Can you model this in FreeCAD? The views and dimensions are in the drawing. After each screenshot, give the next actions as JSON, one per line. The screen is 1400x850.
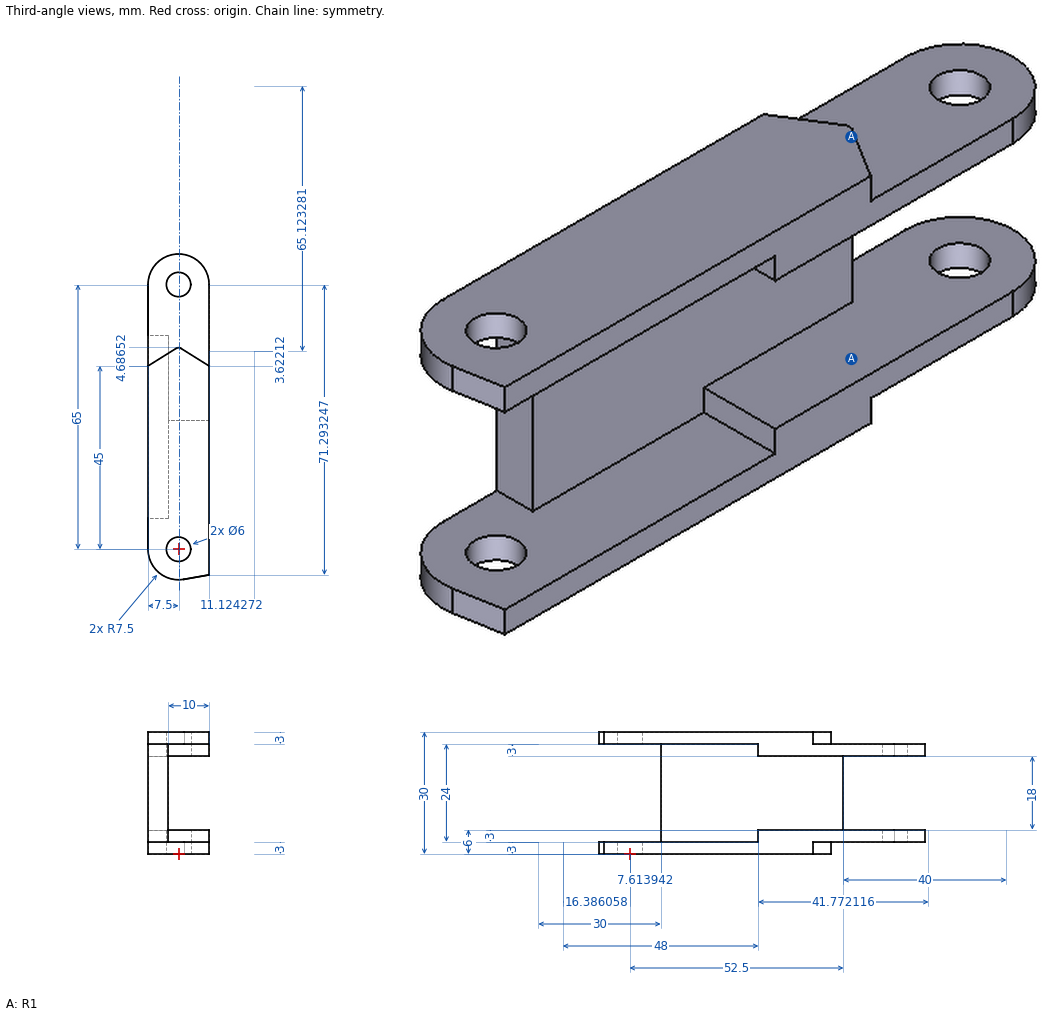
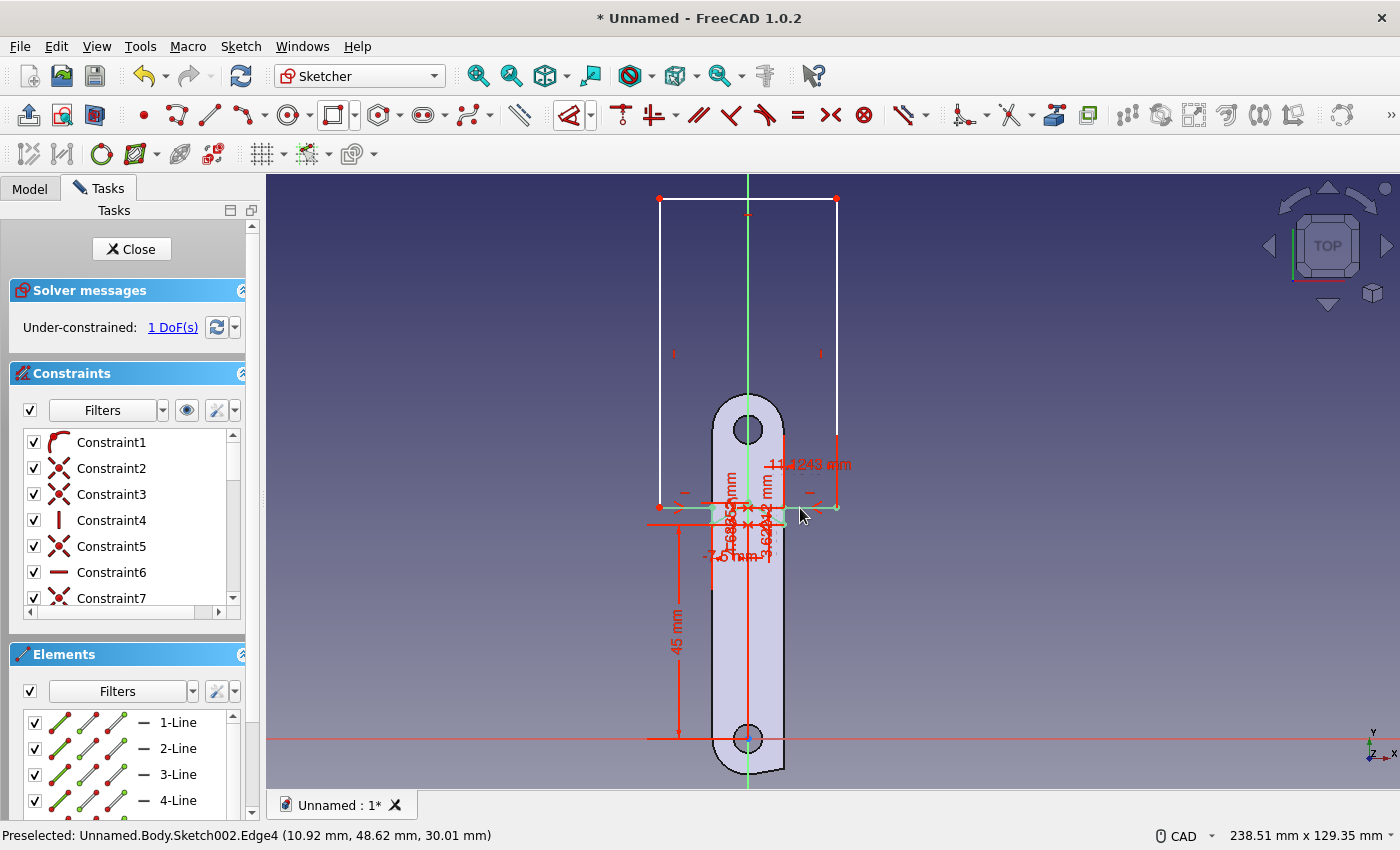
{"action": "left_click", "coordinate": [837, 415]}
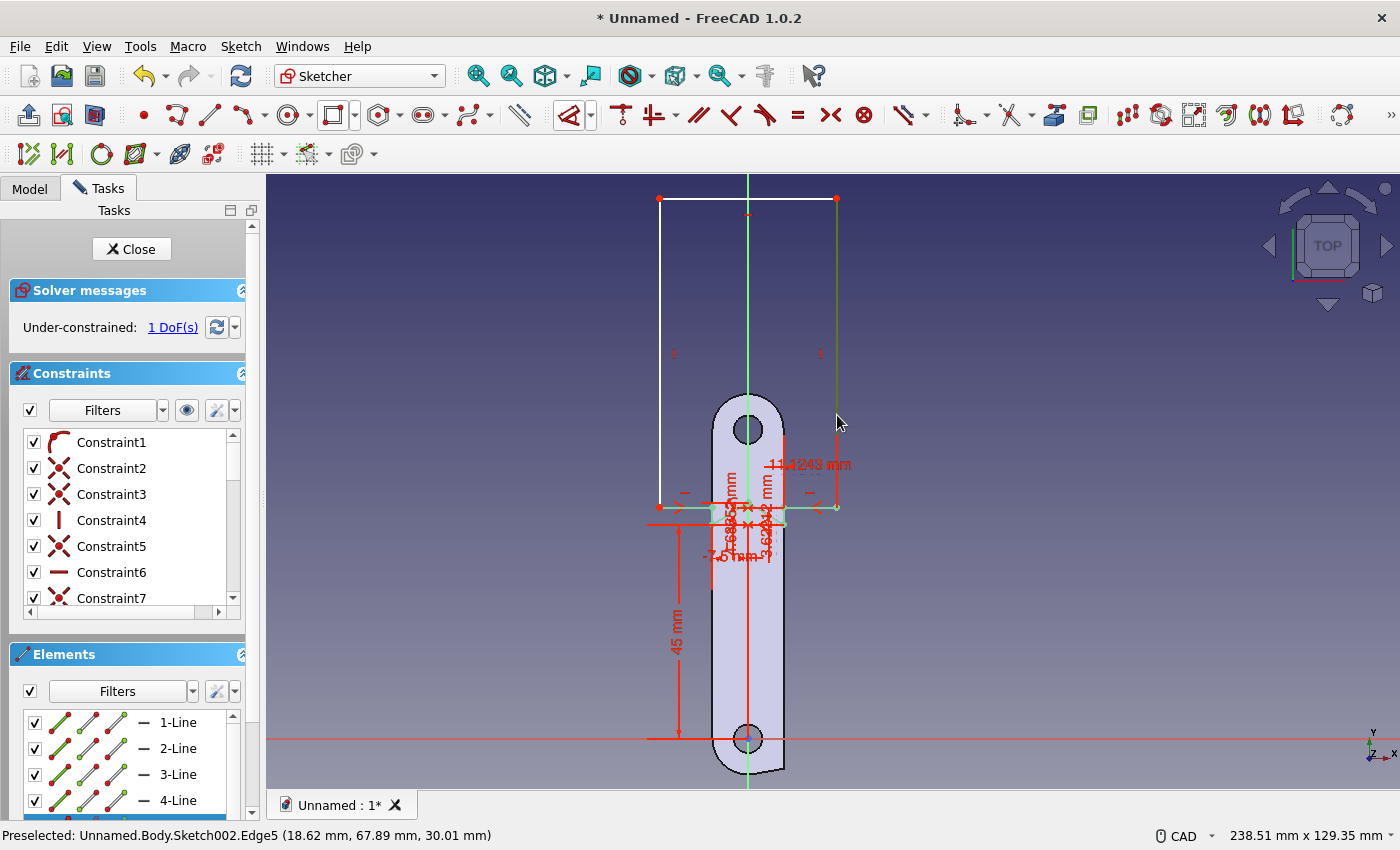
{"action": "left_click", "coordinate": [590, 116]}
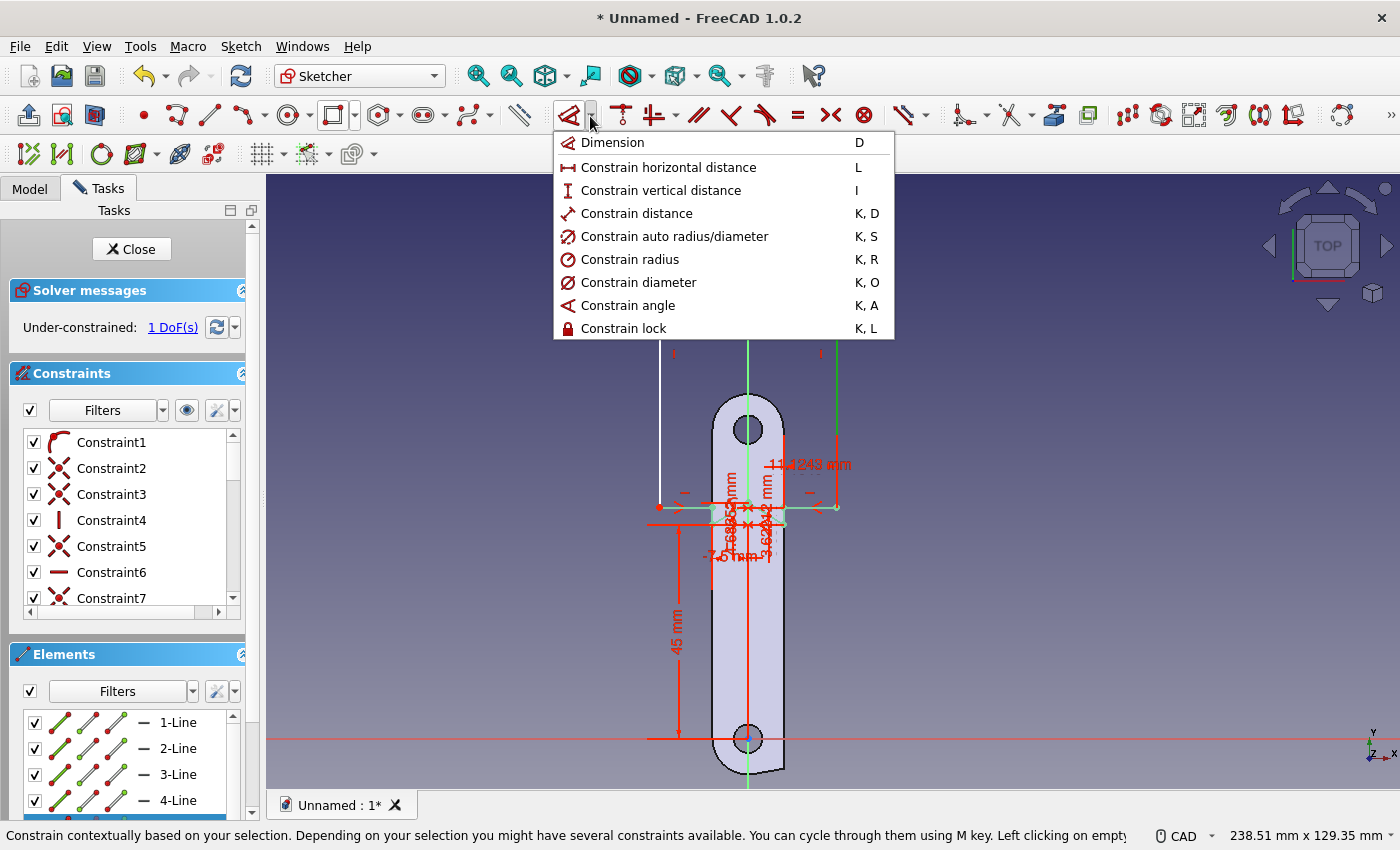
{"action": "left_click", "coordinate": [724, 190]}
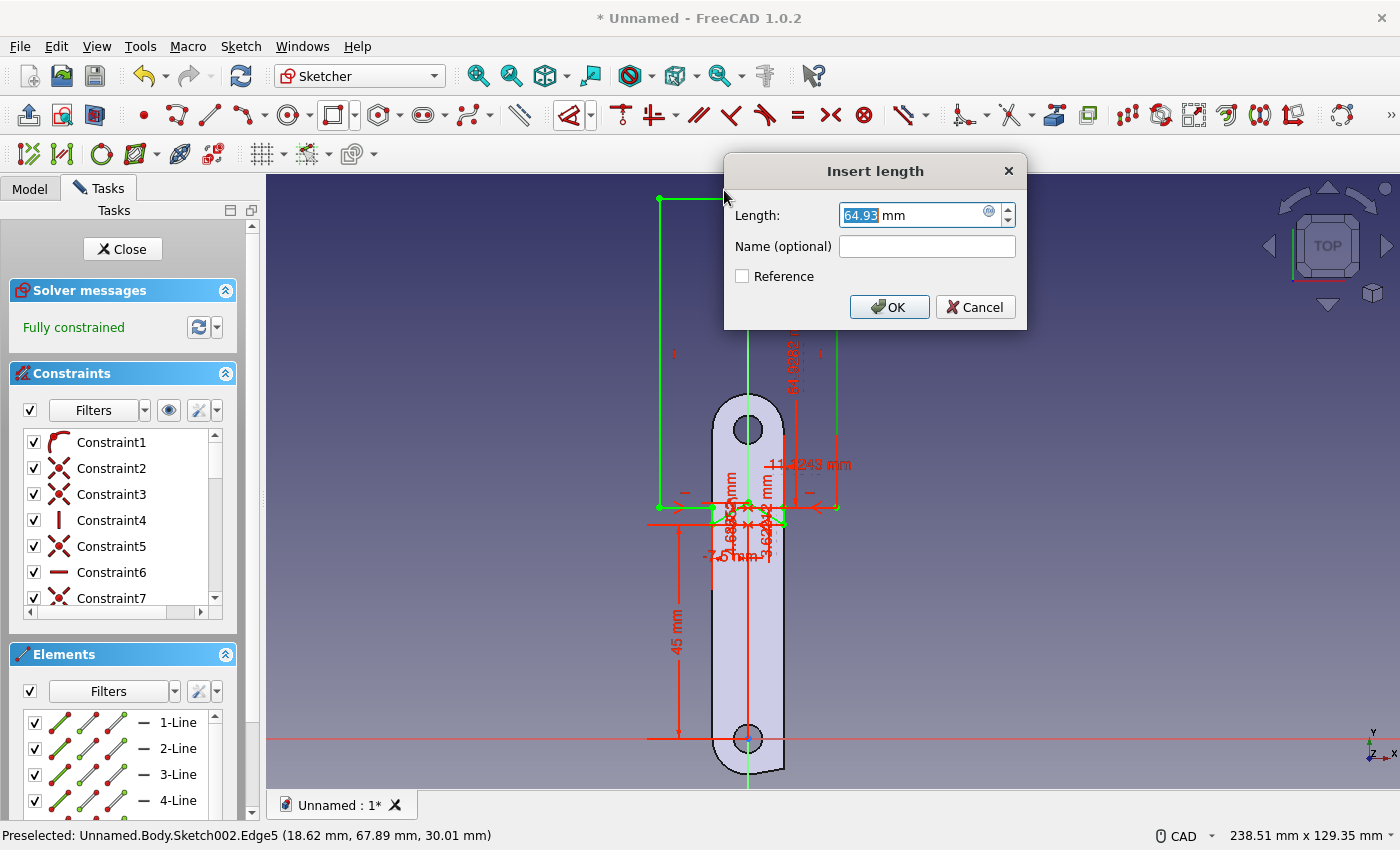
{"action": "type", "text": "65.123281"}
{"action": "key", "text": "Return"}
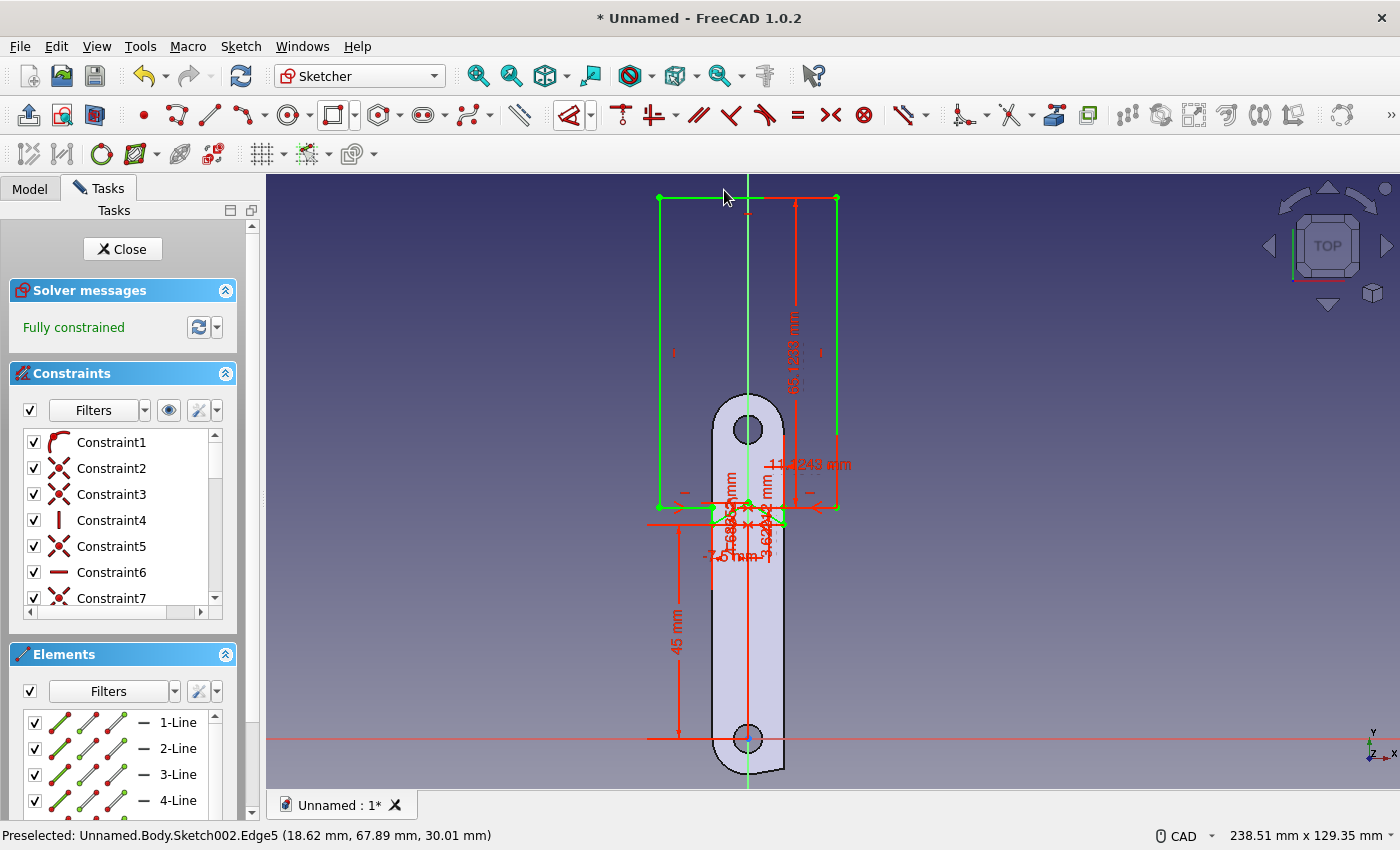
{"action": "left_click", "coordinate": [123, 249]}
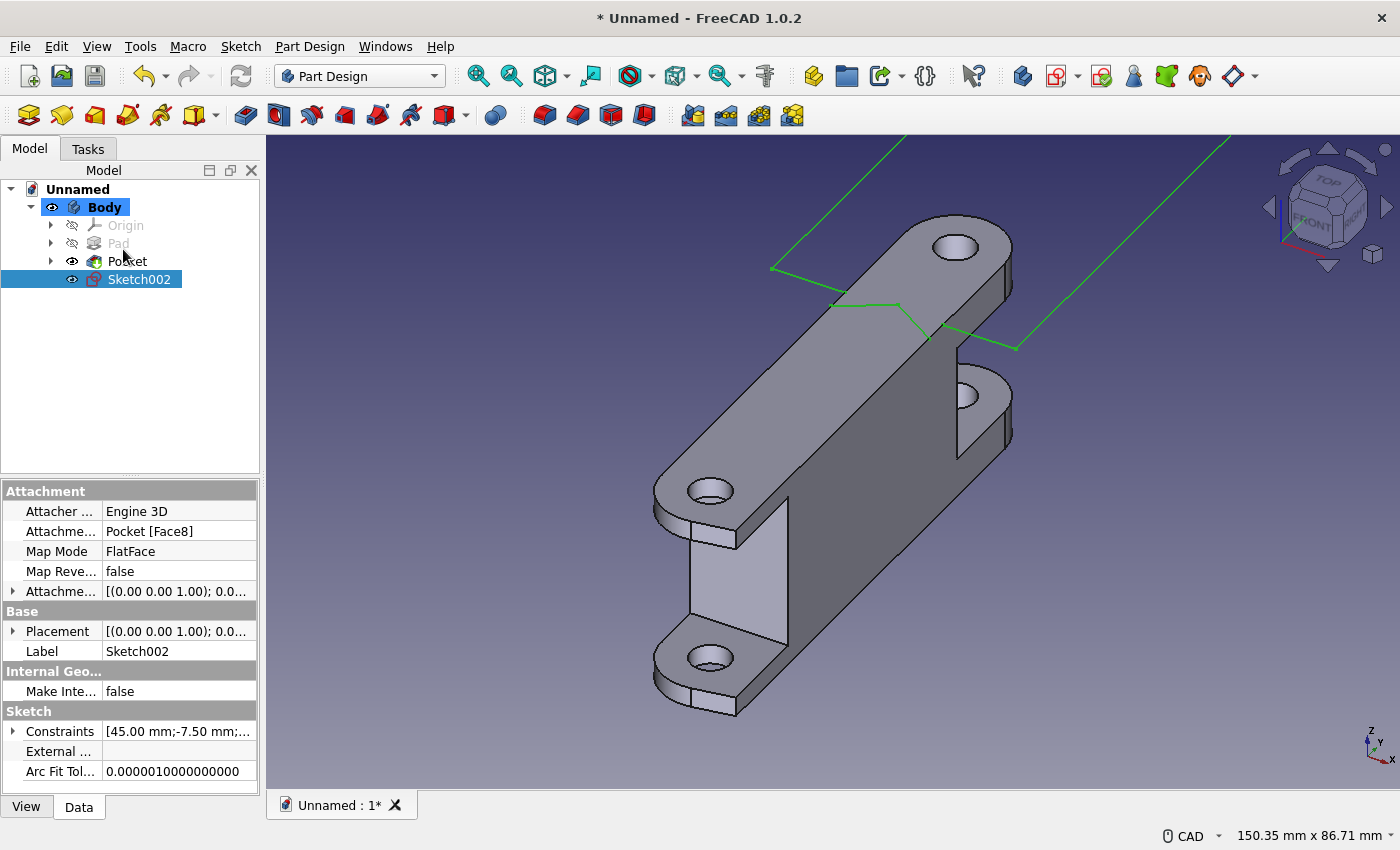
{"action": "left_click", "coordinate": [246, 116]}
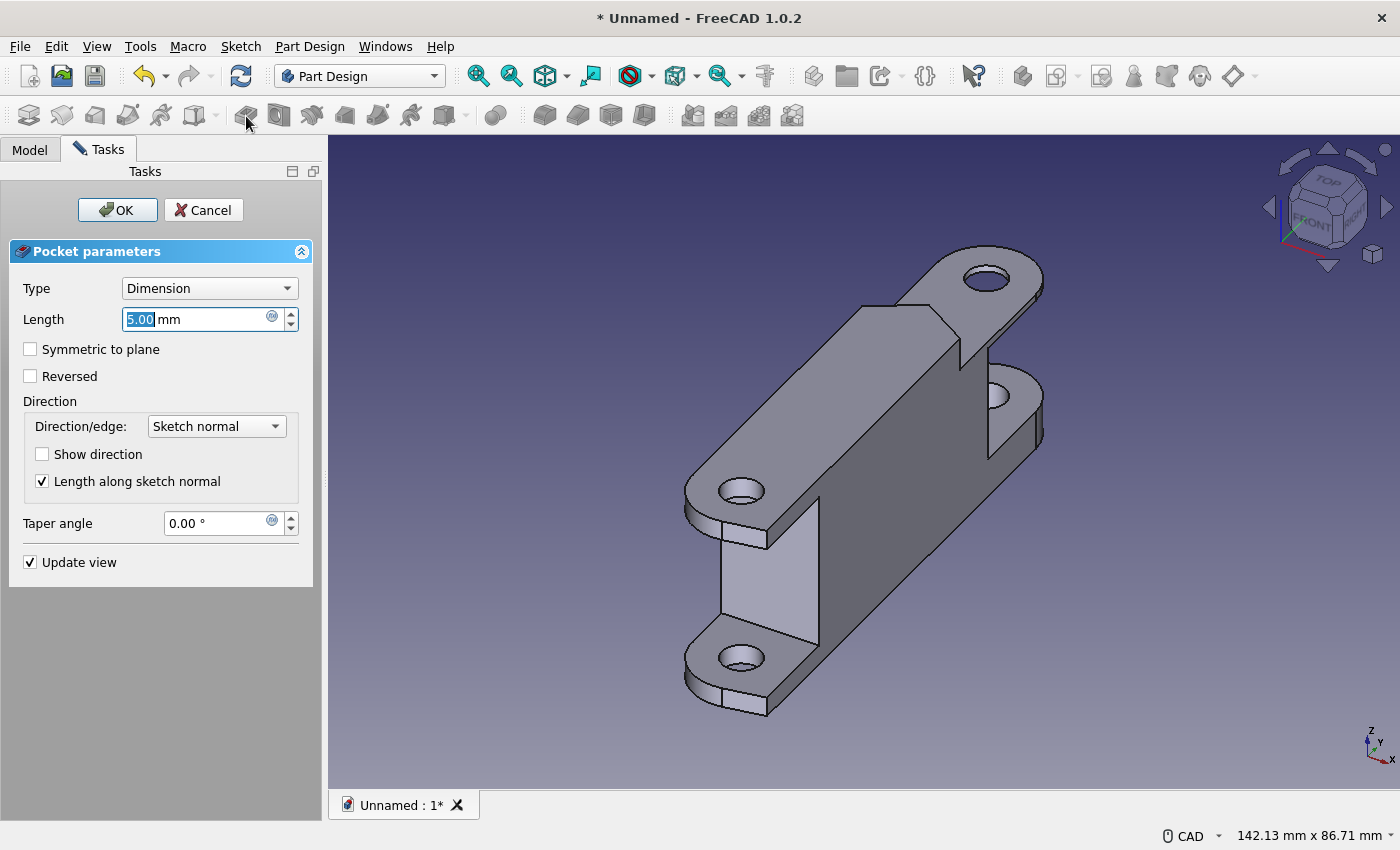
{"action": "type", "text": "3"}
{"action": "key", "text": "Tab"}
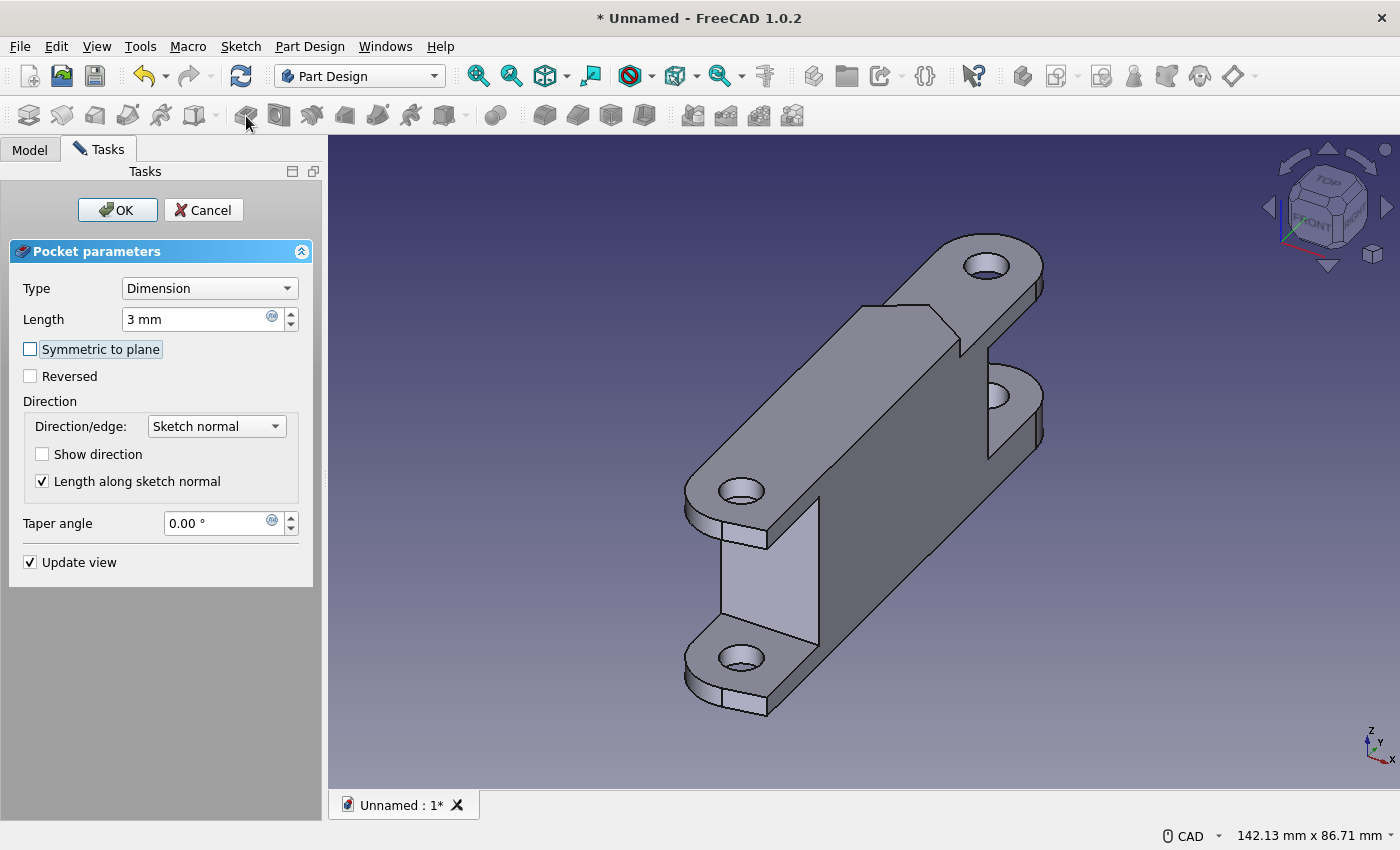
{"action": "left_click", "coordinate": [118, 210]}